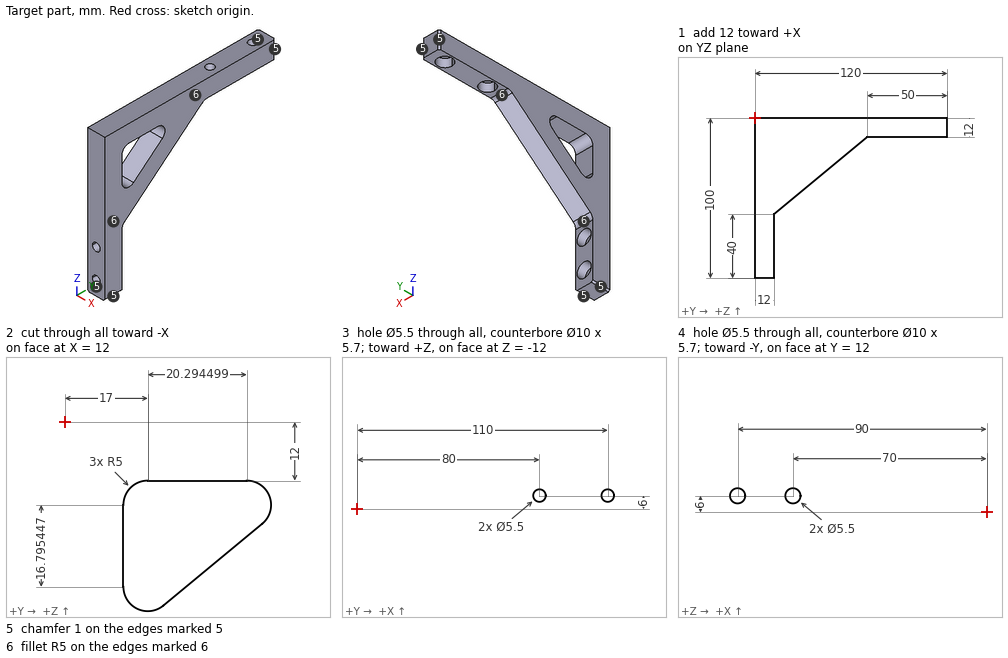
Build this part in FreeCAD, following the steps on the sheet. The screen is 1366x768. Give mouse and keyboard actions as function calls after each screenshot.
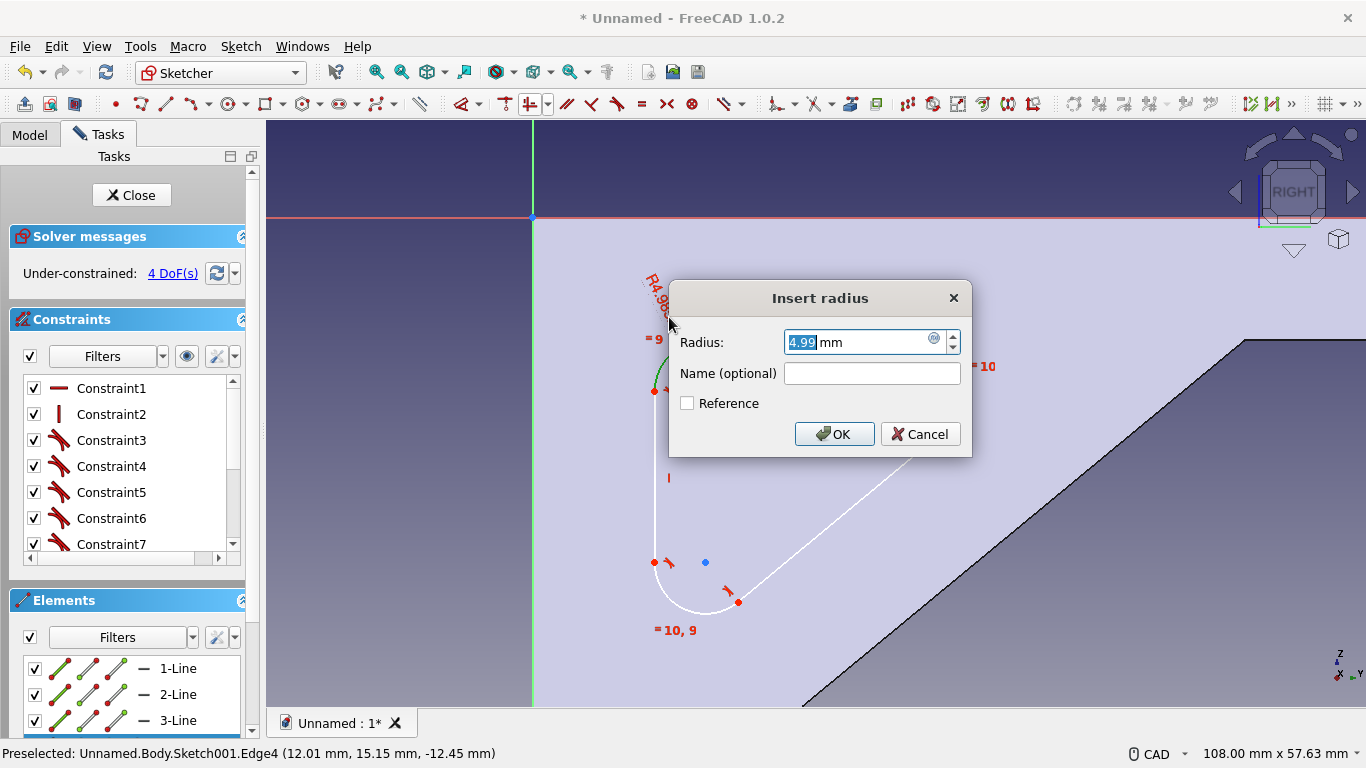
text(5)
key(Return)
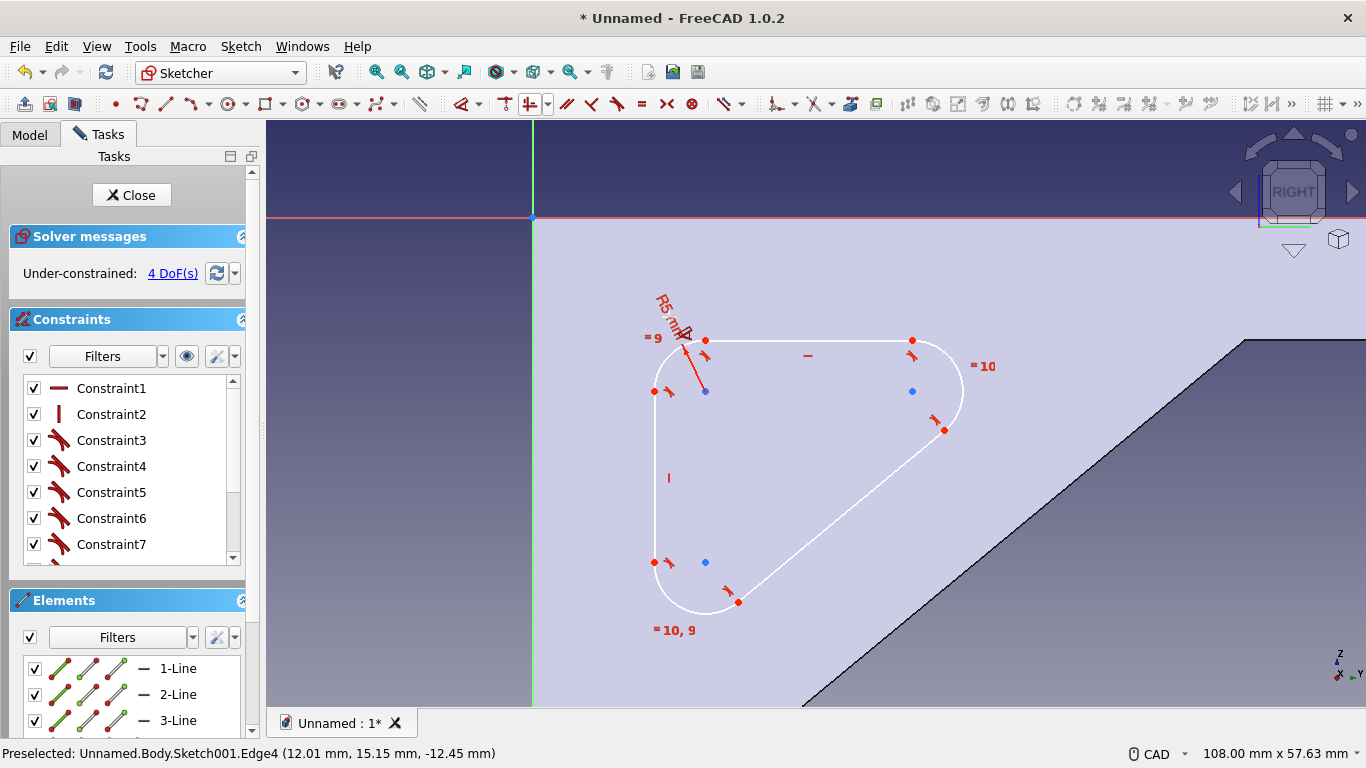
click(912, 341)
click(499, 279)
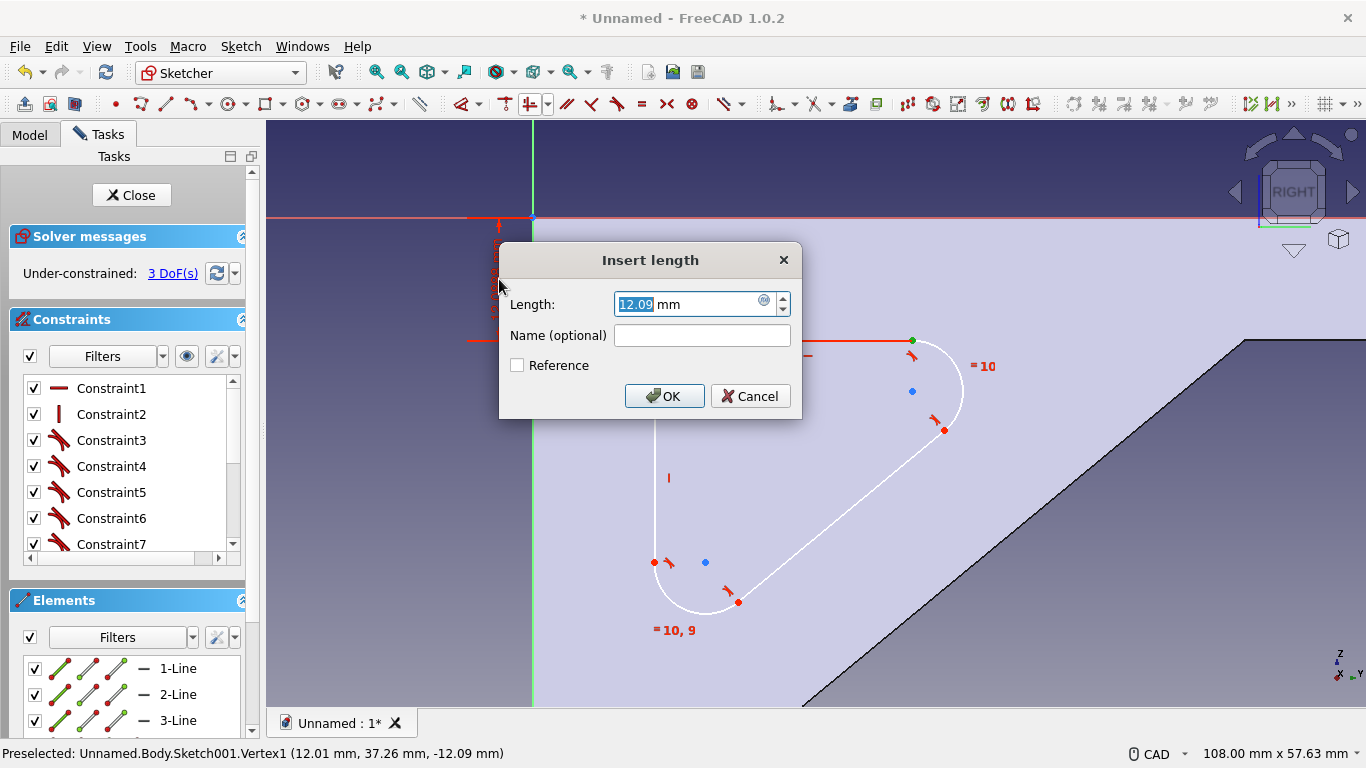
text(12)
key(Return)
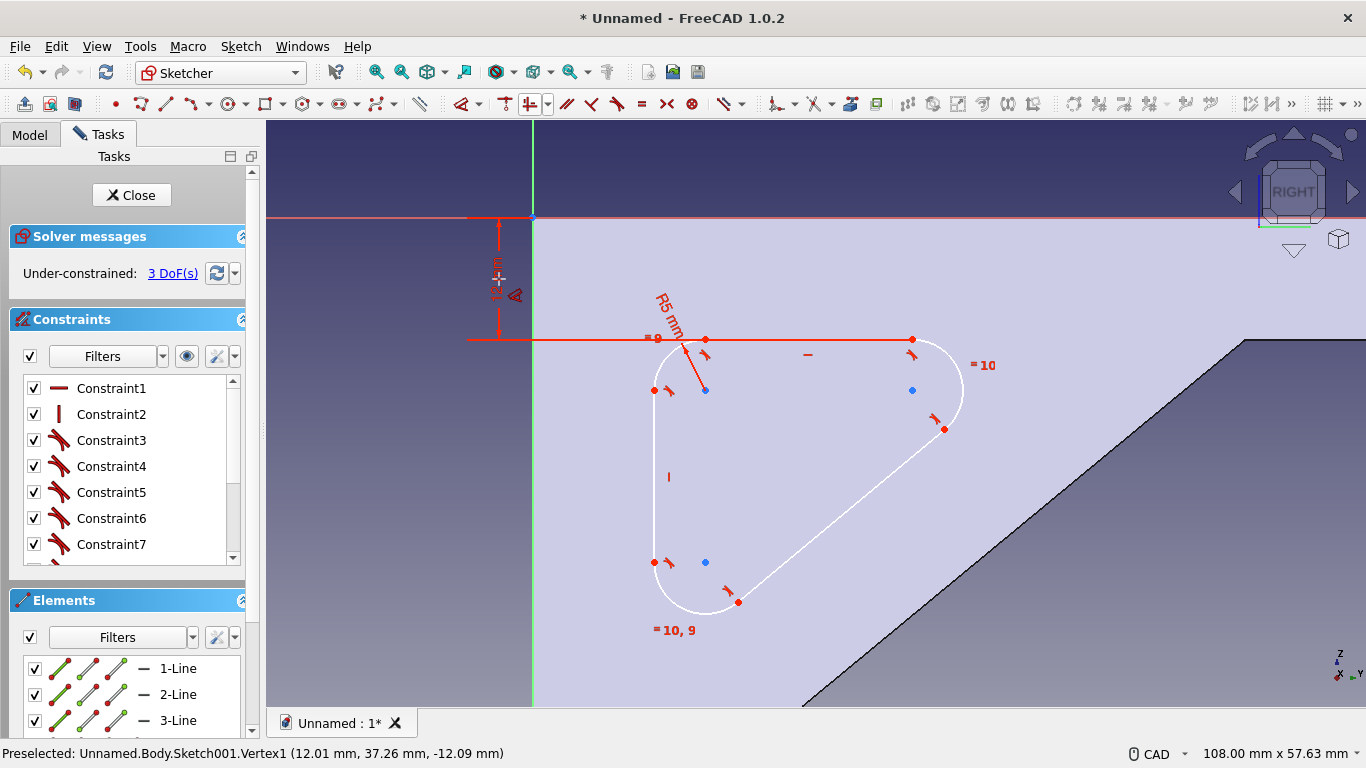
click(705, 340)
click(619, 184)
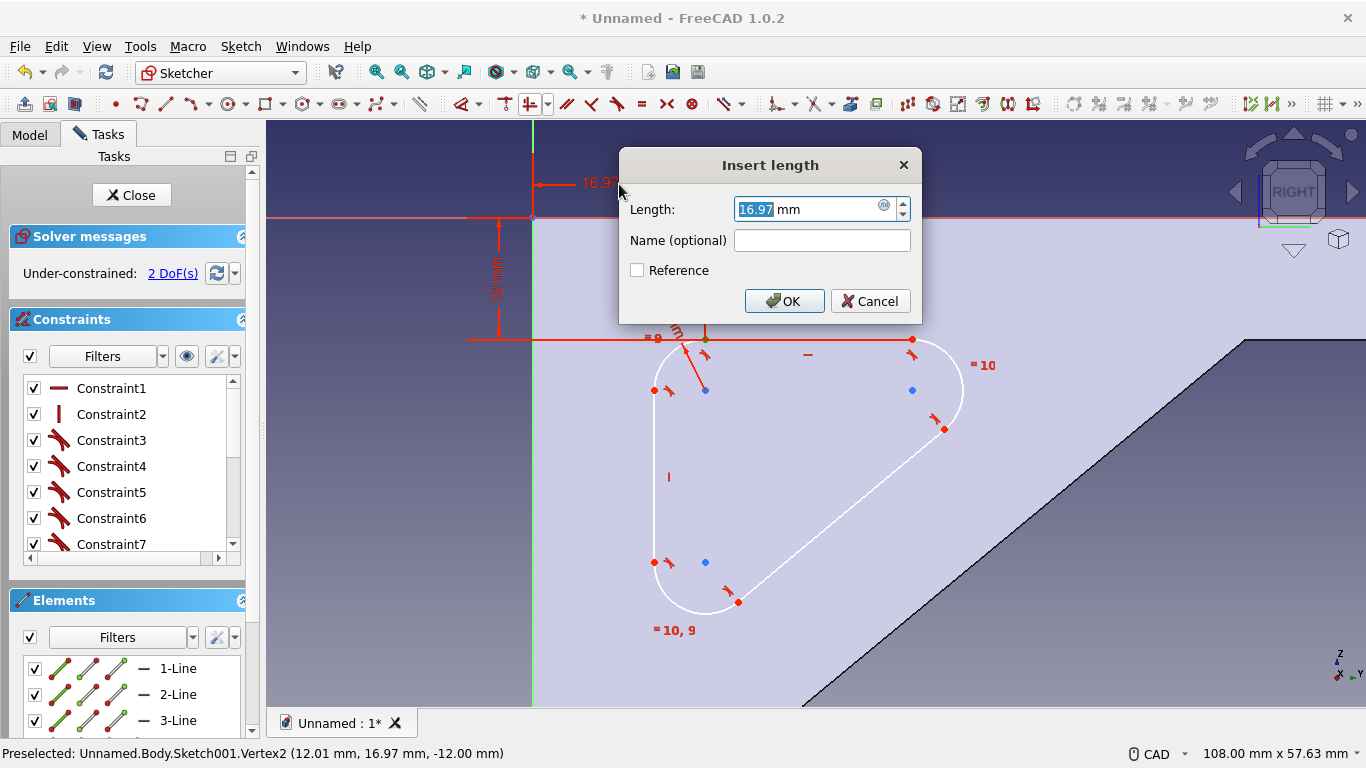
text(17)
key(Return)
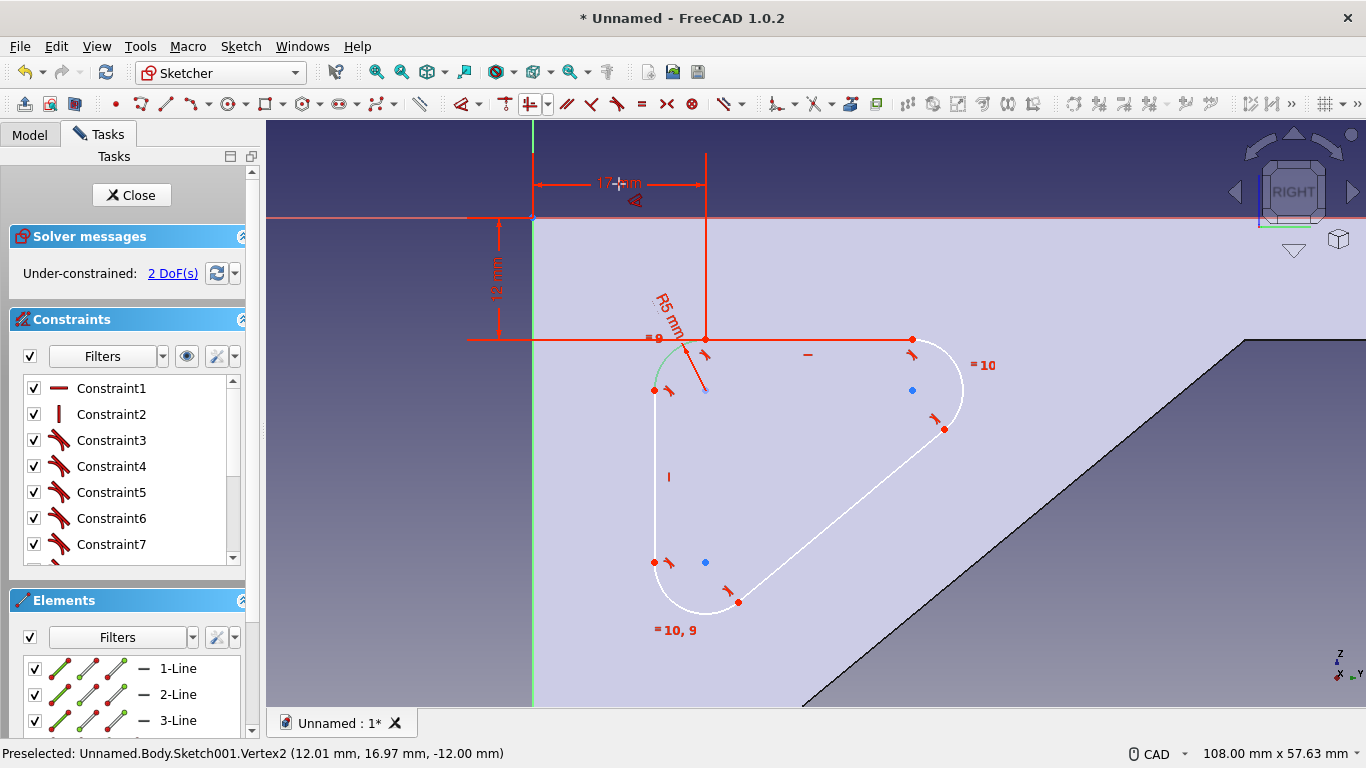
click(850, 340)
click(809, 306)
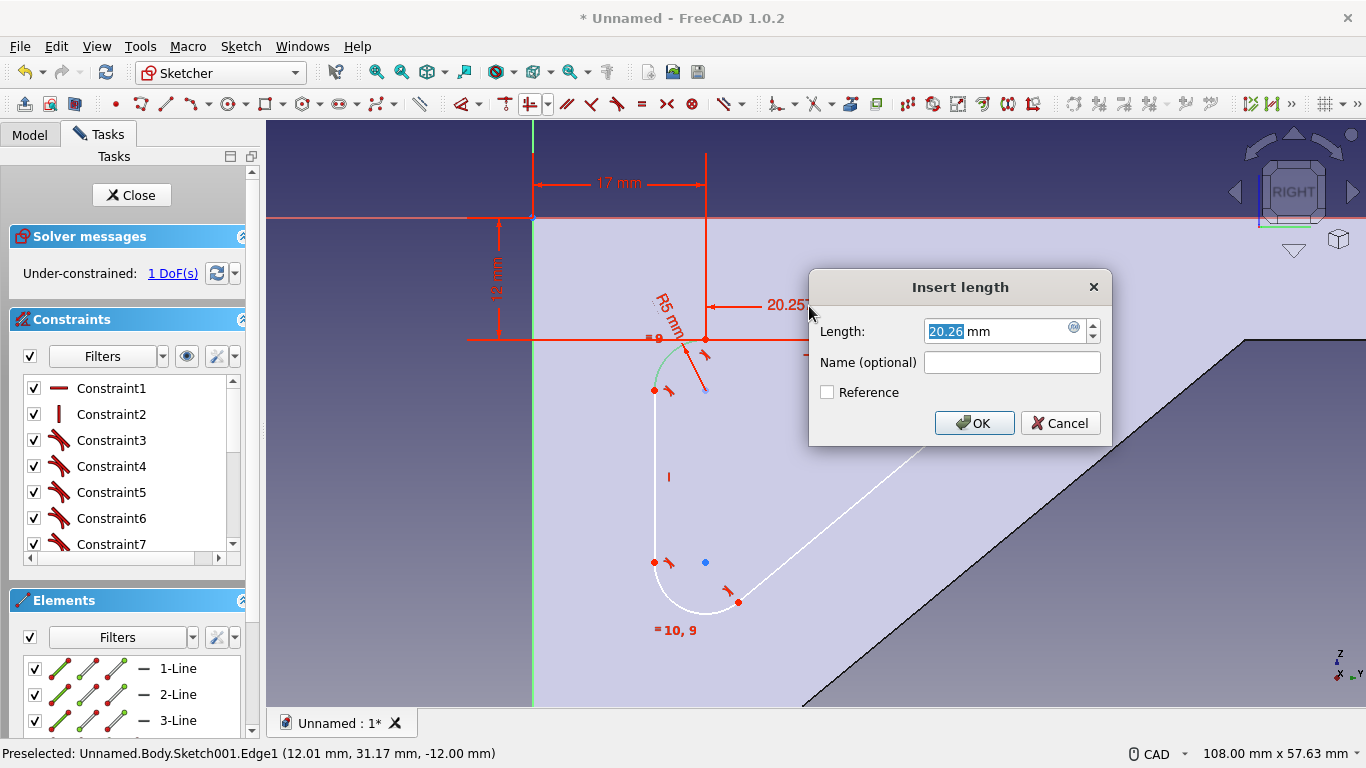
text(20.294499)
key(Return)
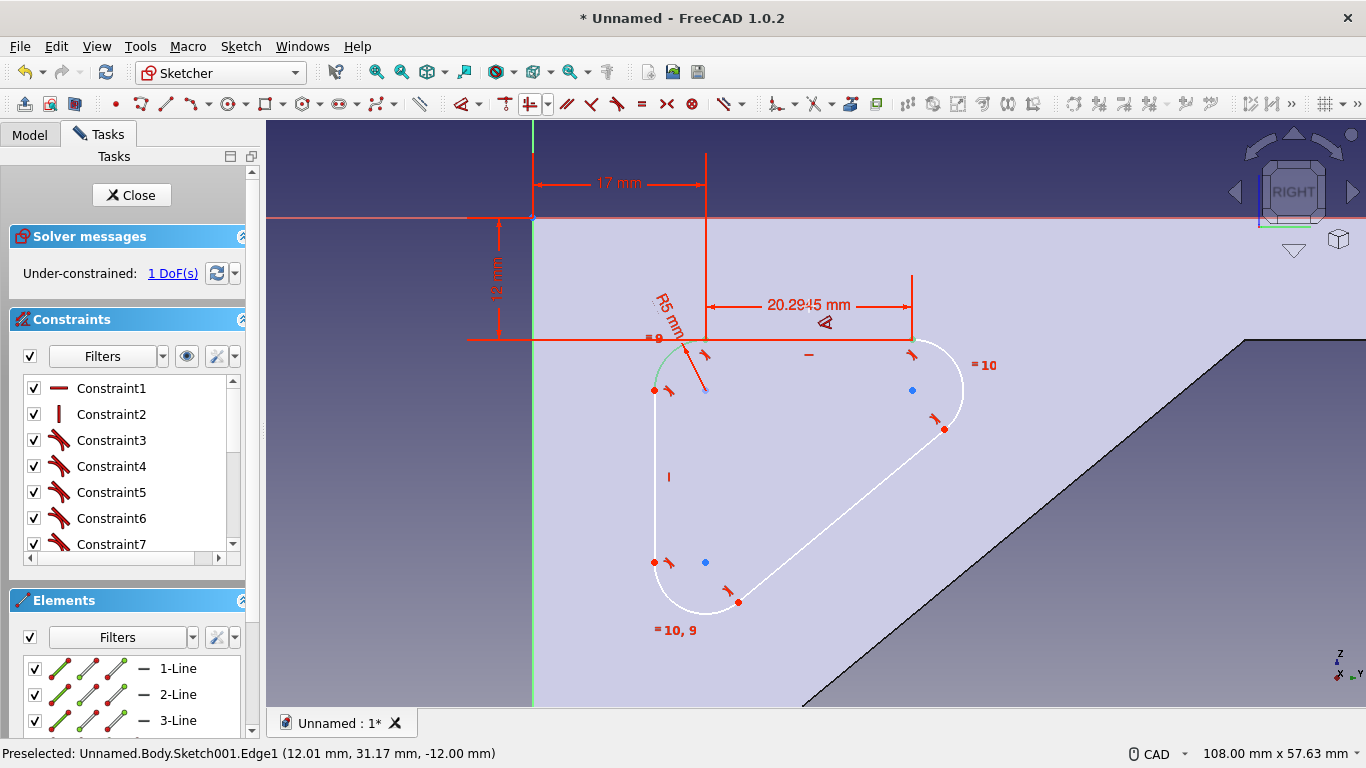
click(655, 442)
click(621, 477)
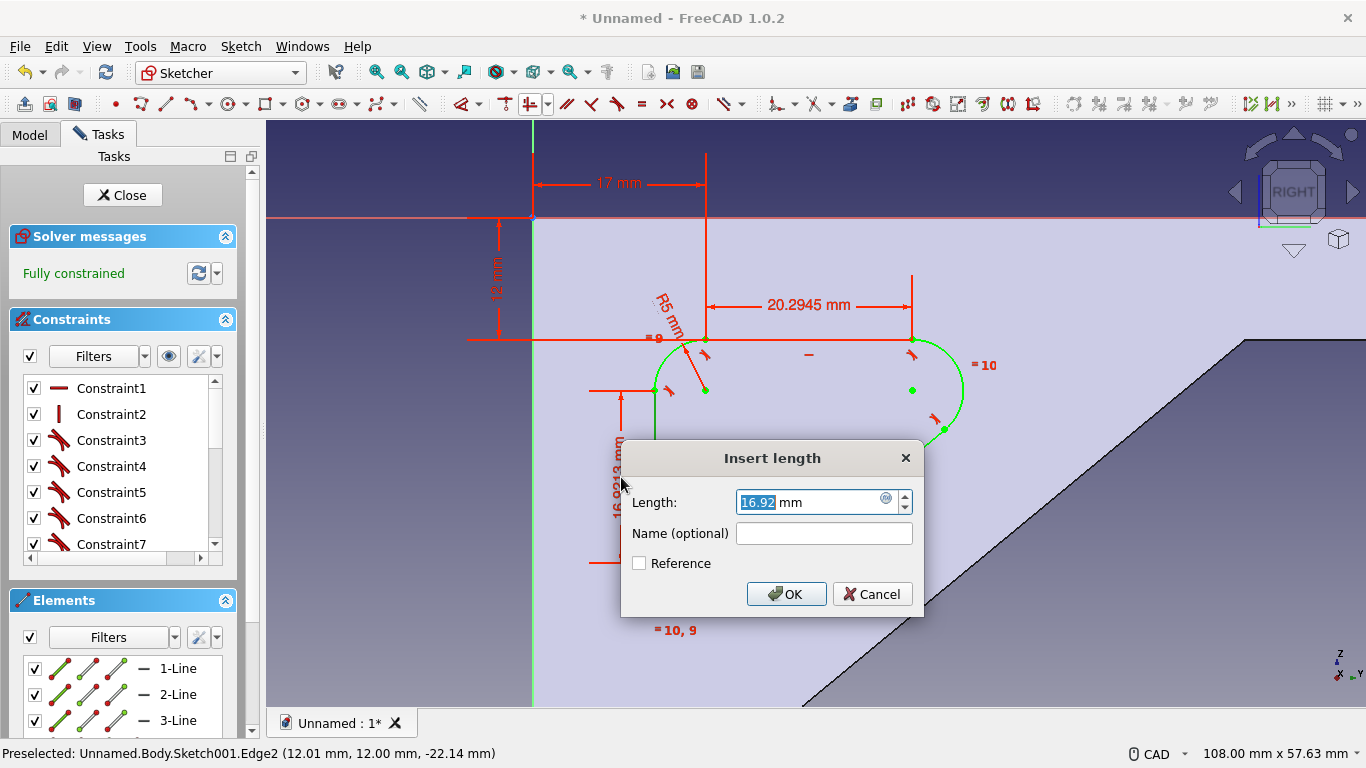
text(16.795447)
key(Return)
key(Escape)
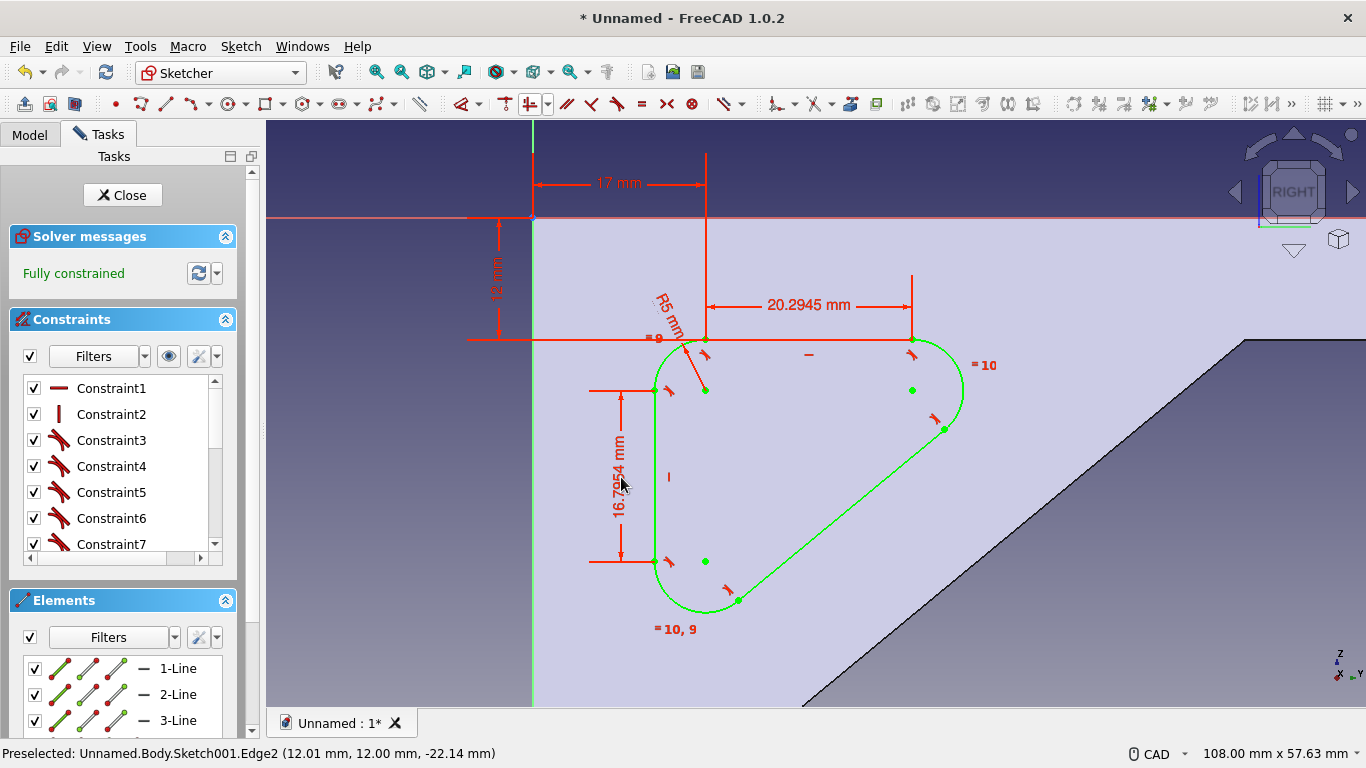
click(123, 195)